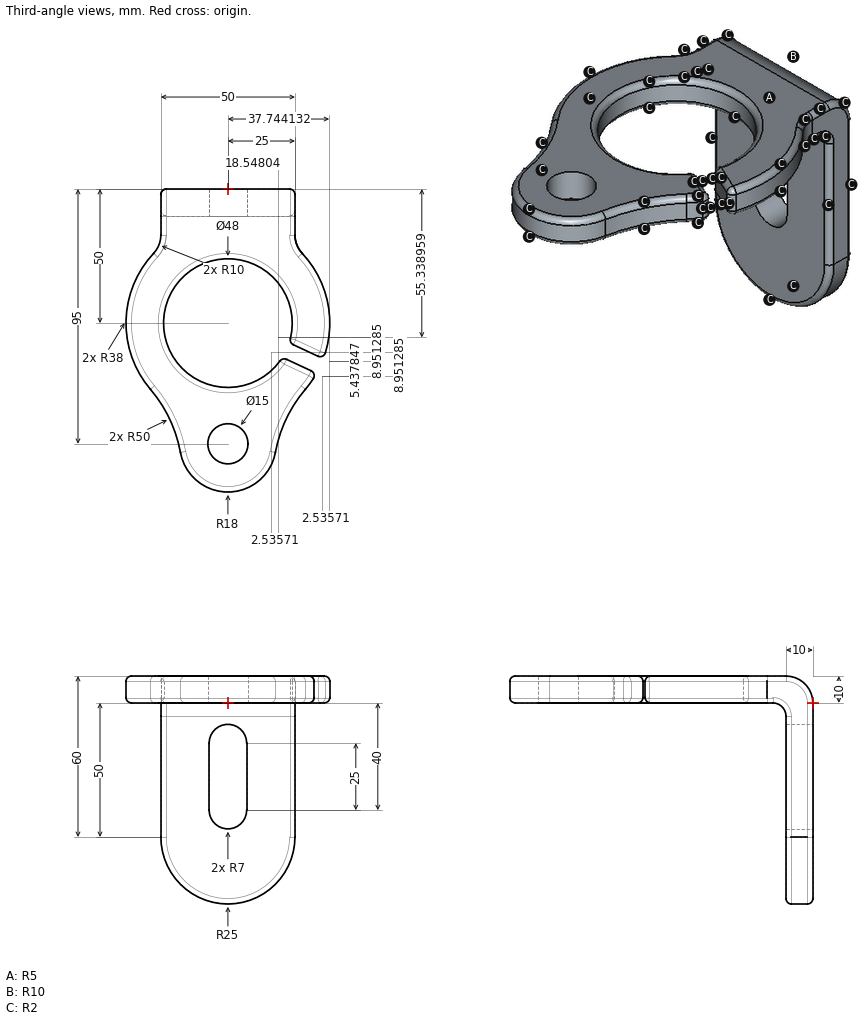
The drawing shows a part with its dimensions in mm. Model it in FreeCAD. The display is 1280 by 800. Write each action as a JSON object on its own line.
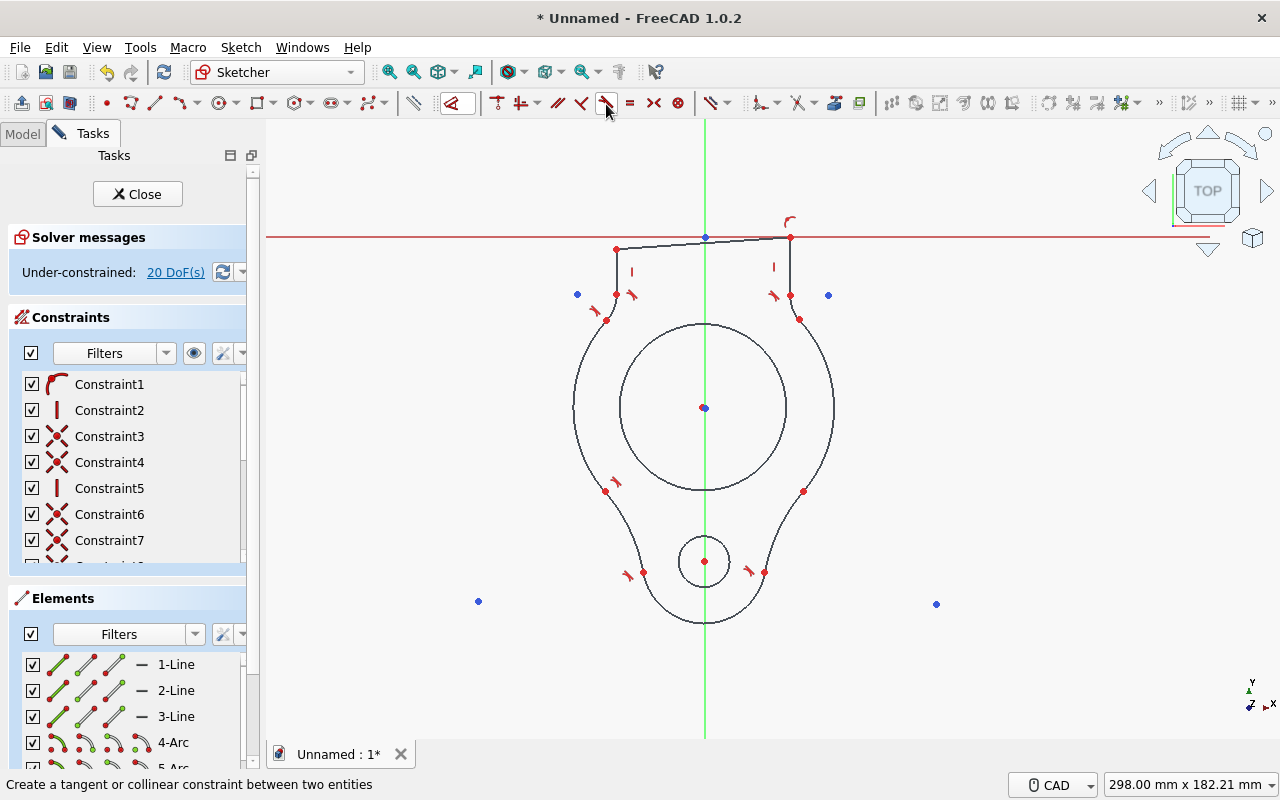
{"action": "left_click", "coordinate": [787, 514]}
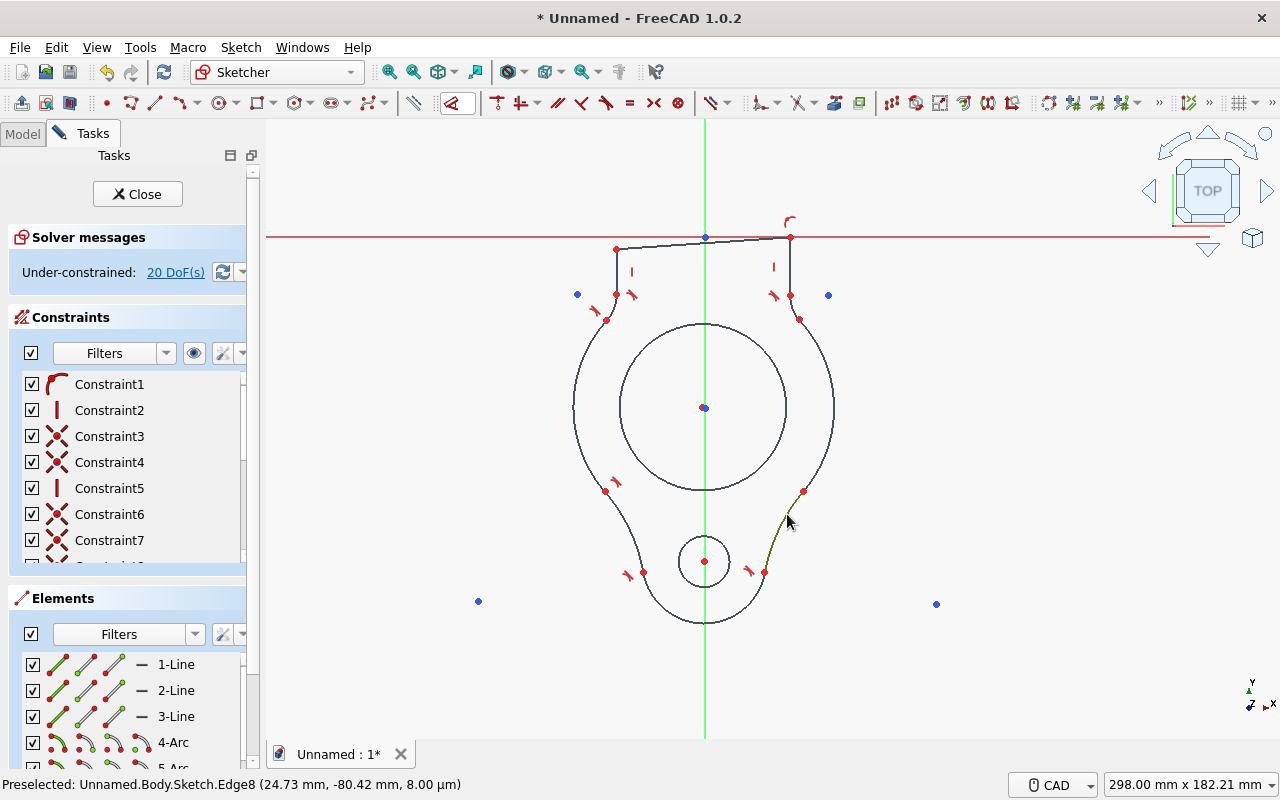
{"action": "left_click", "coordinate": [829, 443]}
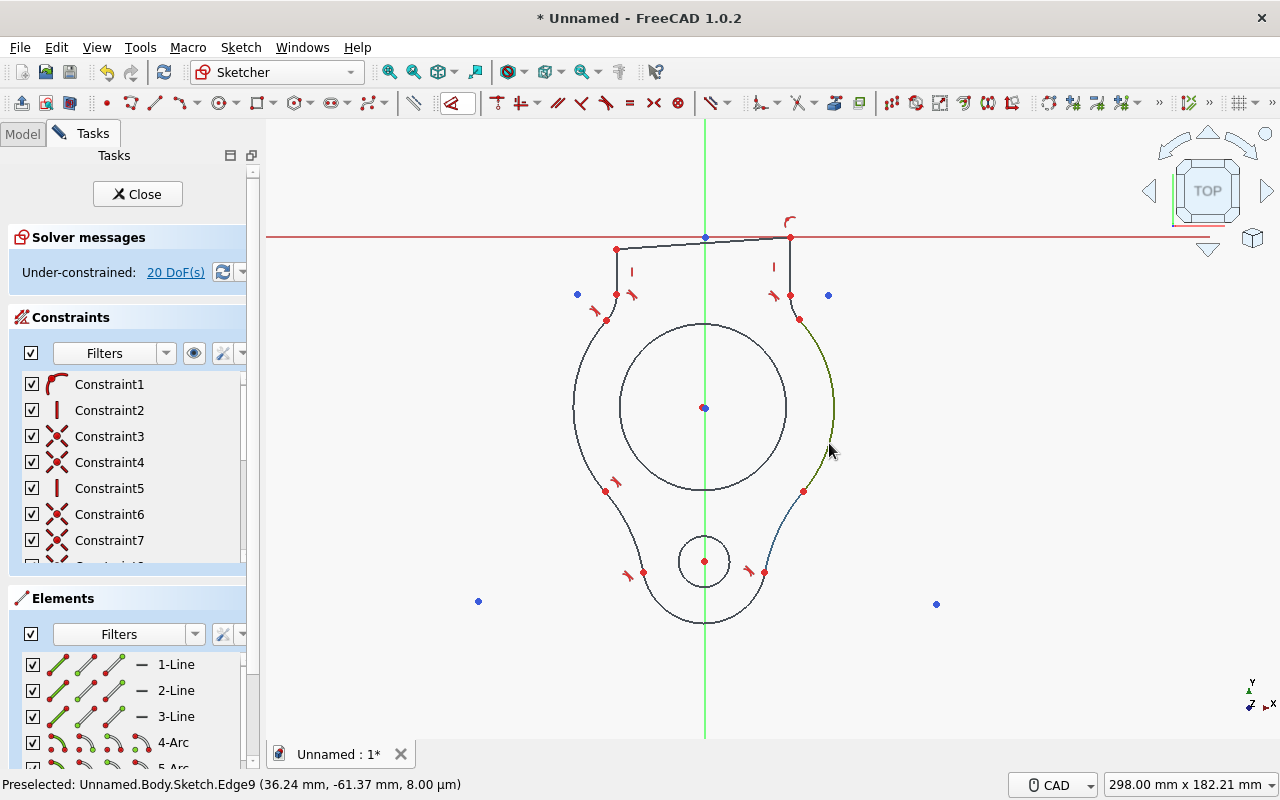
{"action": "left_click", "coordinate": [606, 104]}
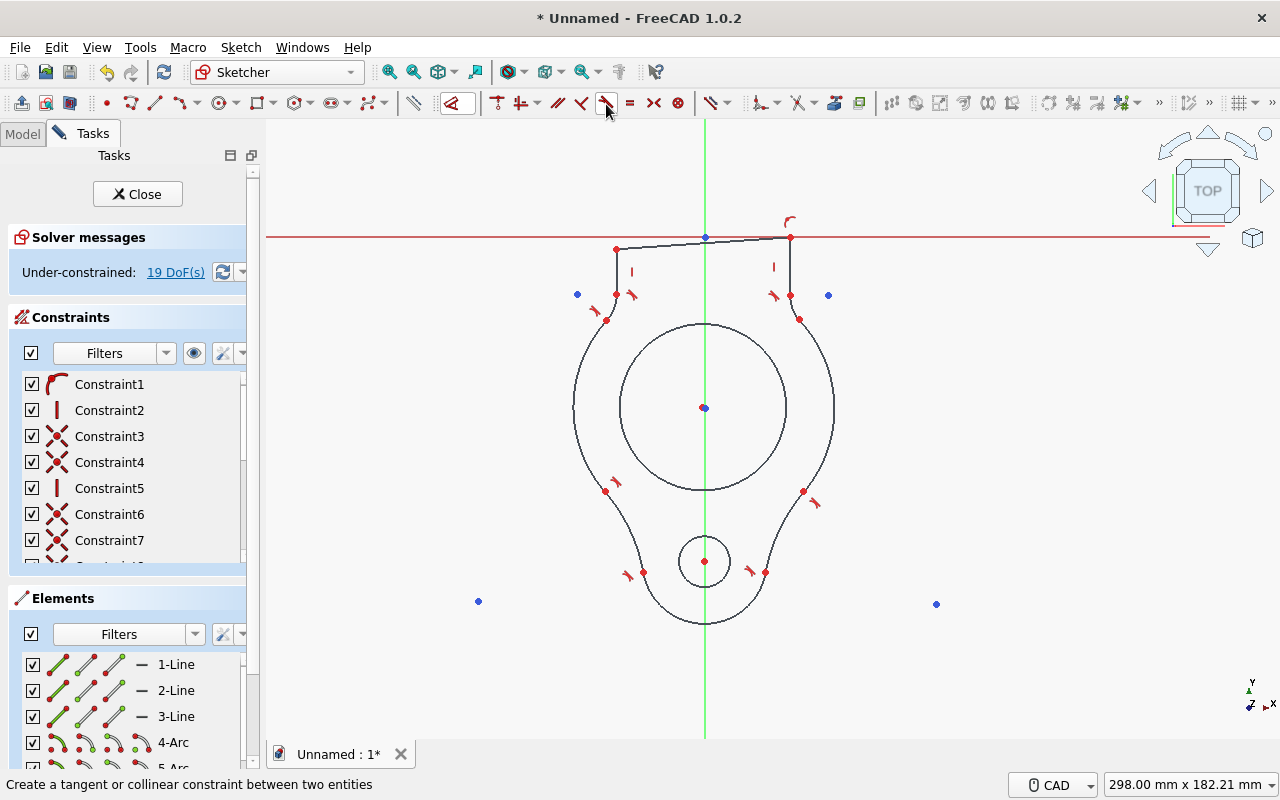
{"action": "left_click", "coordinate": [830, 442]}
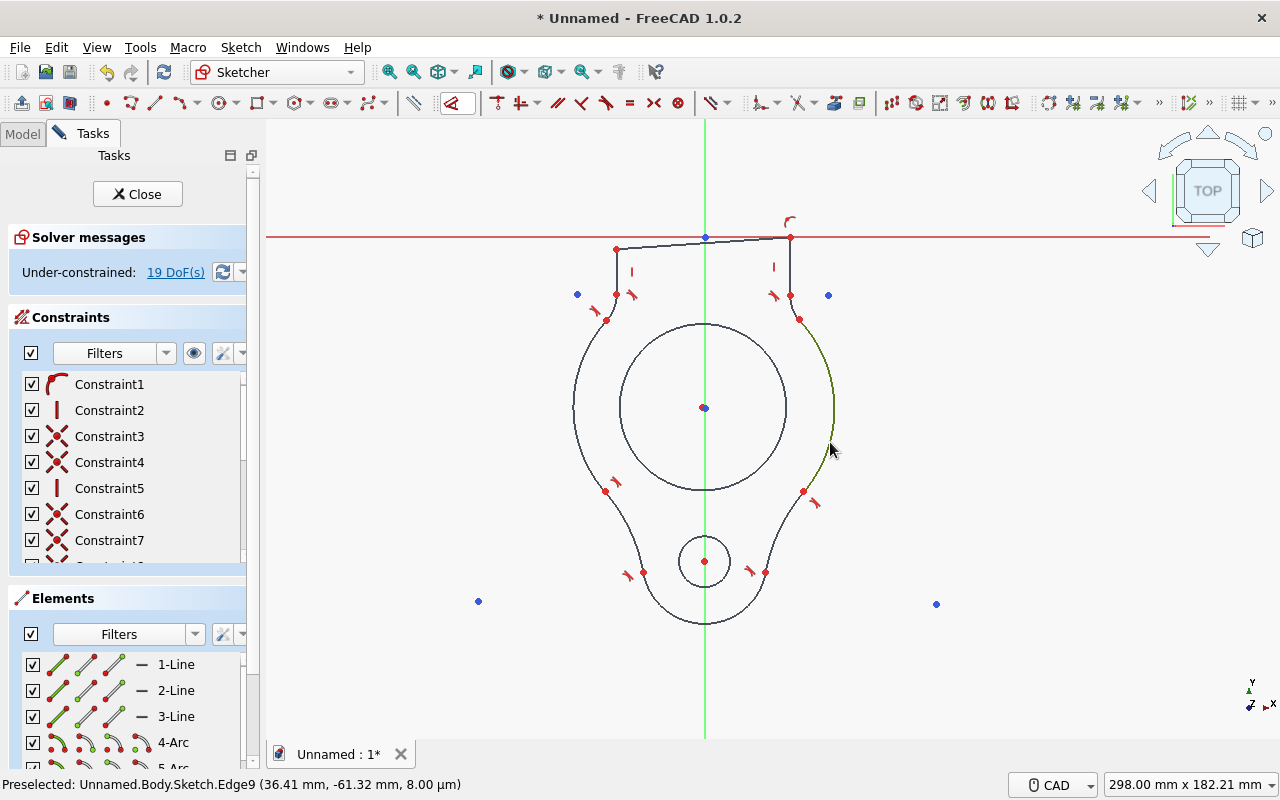
{"action": "left_click", "coordinate": [793, 309]}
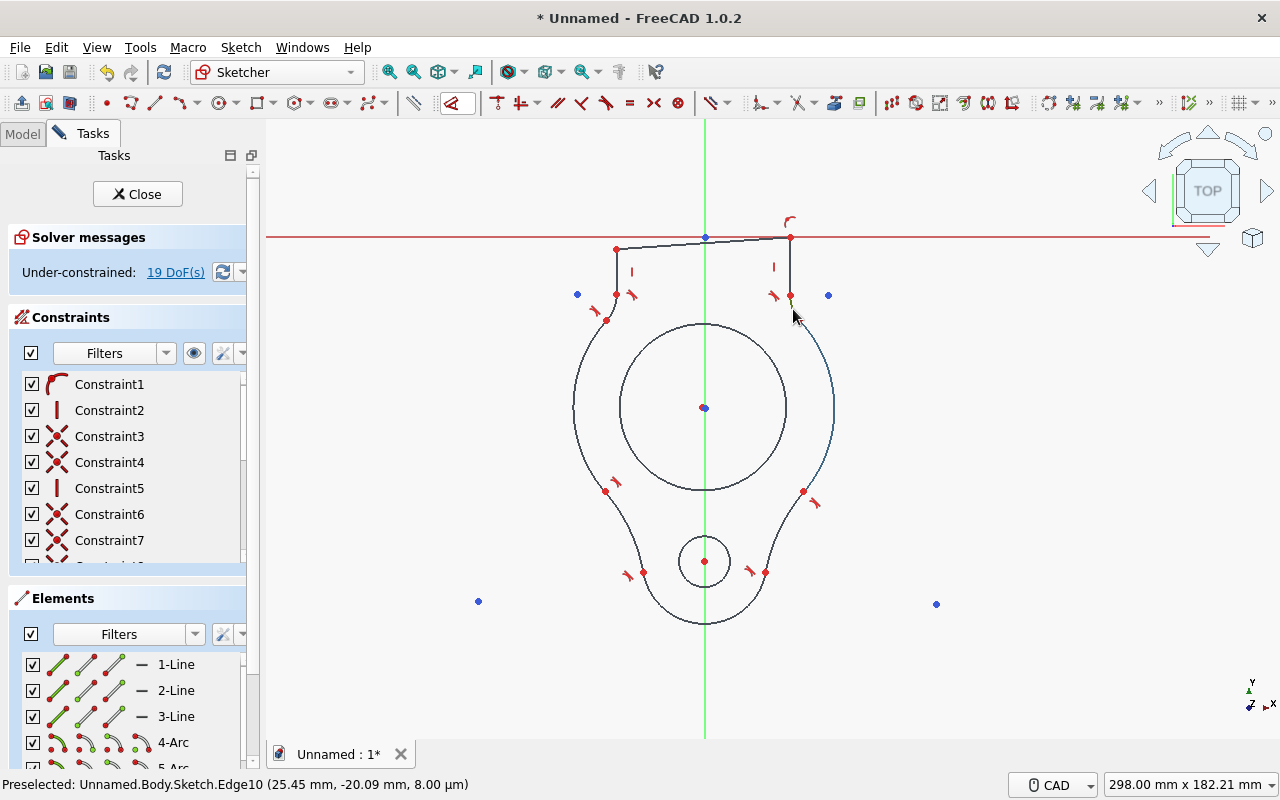
{"action": "left_click", "coordinate": [606, 104]}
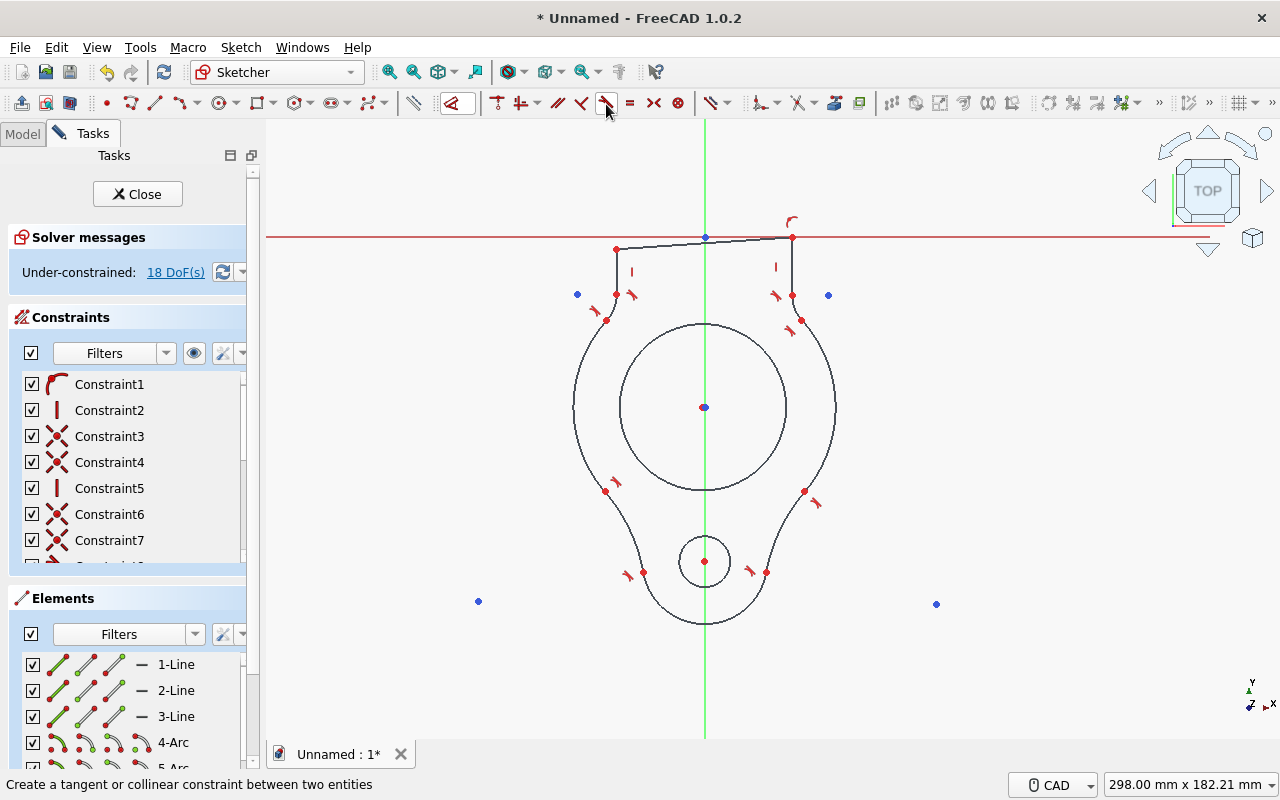
{"action": "left_click", "coordinate": [740, 241]}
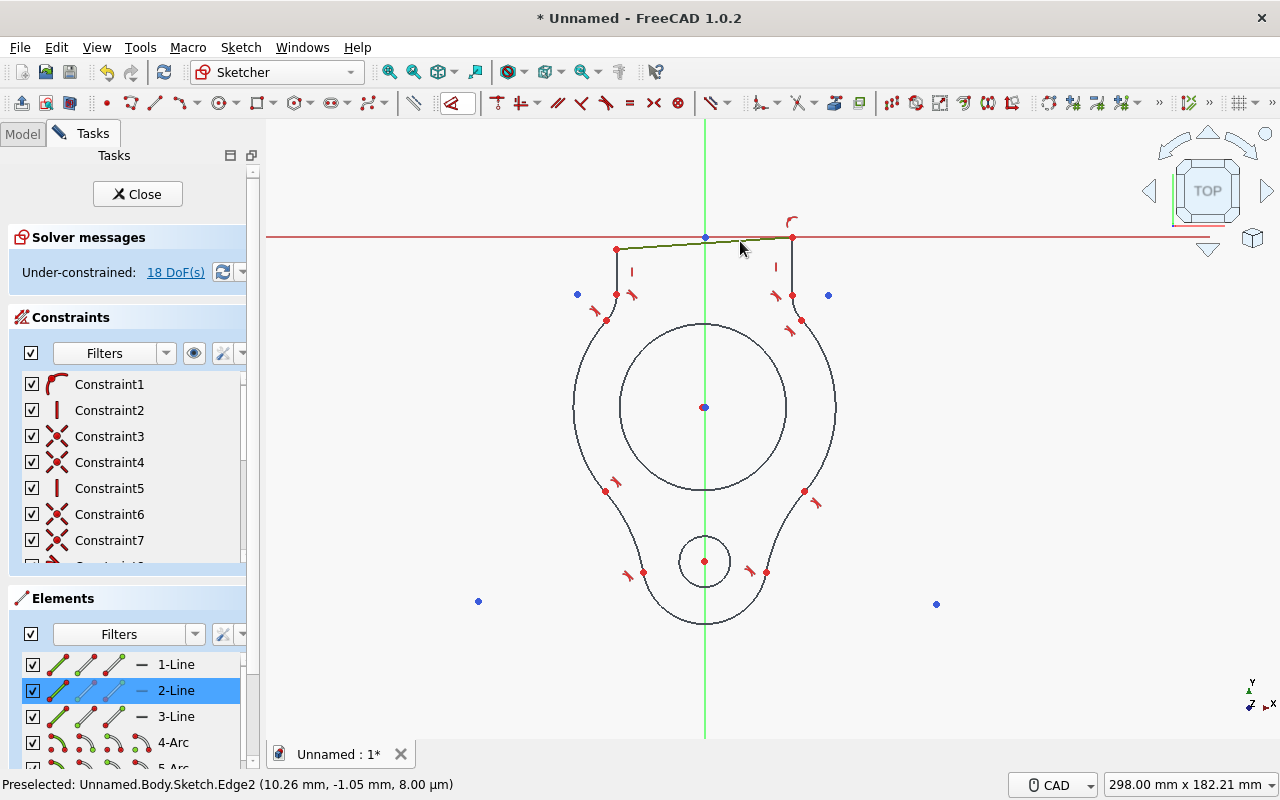
{"action": "key", "text": "h"}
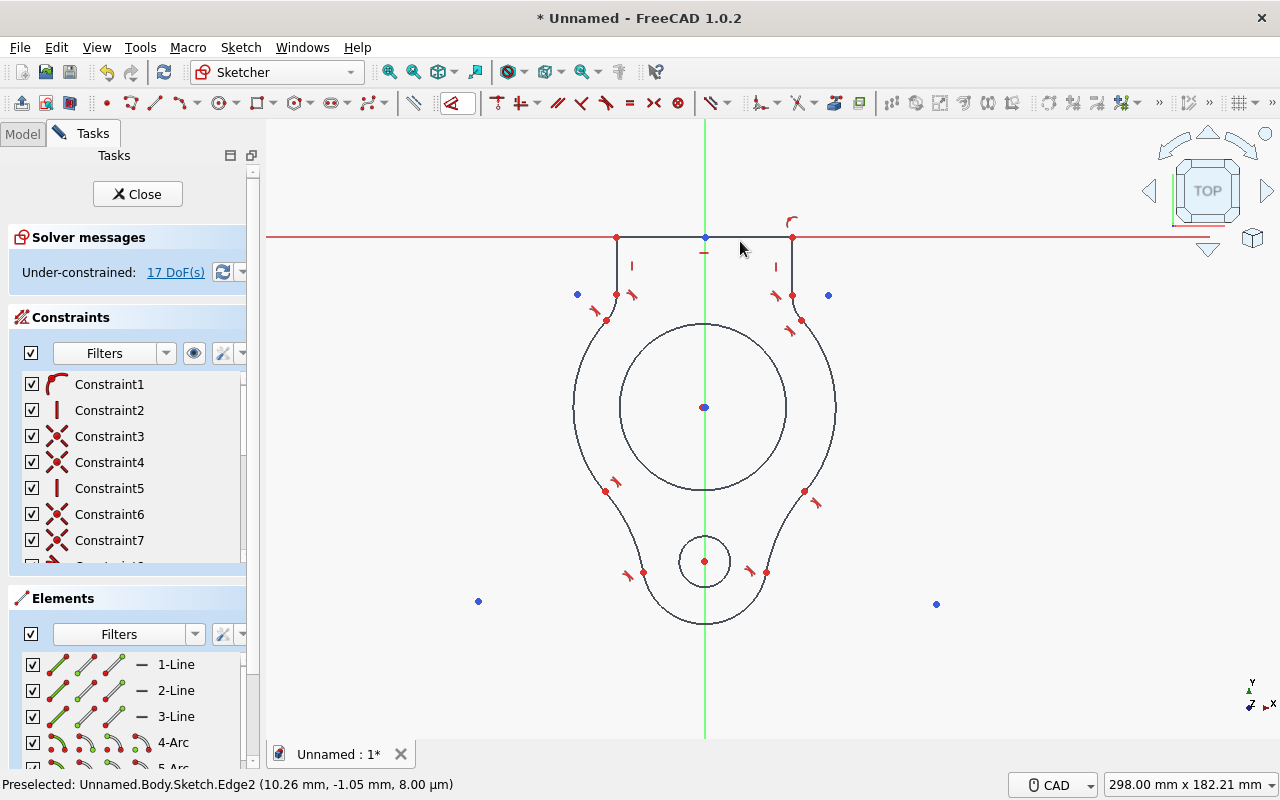
{"action": "left_click", "coordinate": [762, 348]}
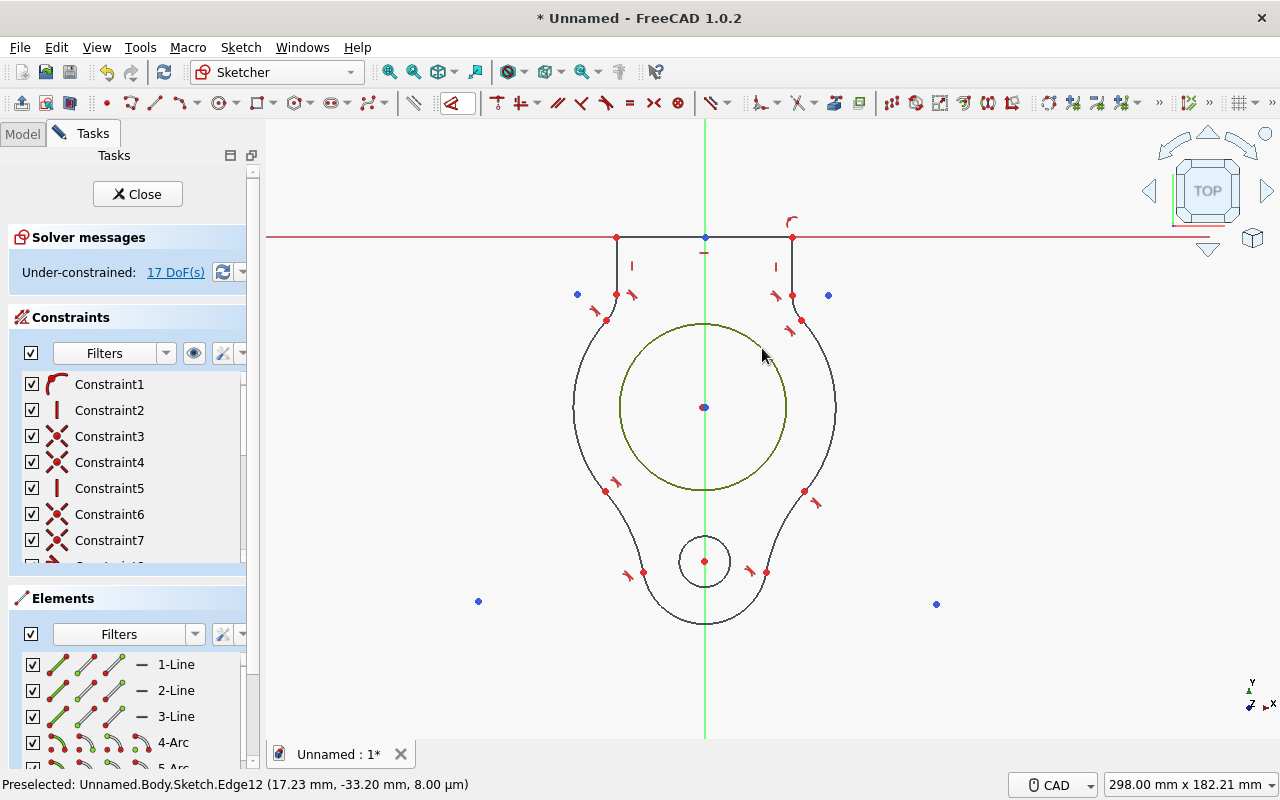
{"action": "left_click", "coordinate": [831, 443]}